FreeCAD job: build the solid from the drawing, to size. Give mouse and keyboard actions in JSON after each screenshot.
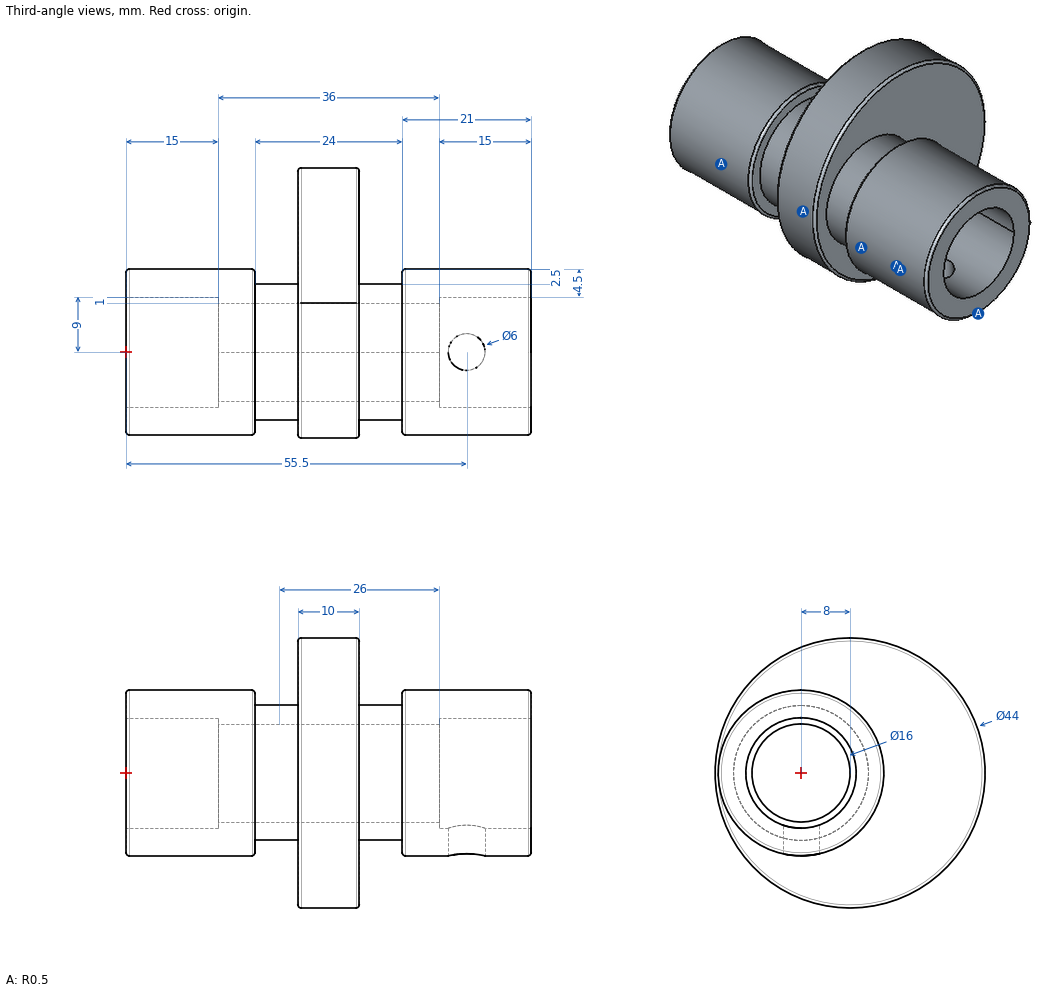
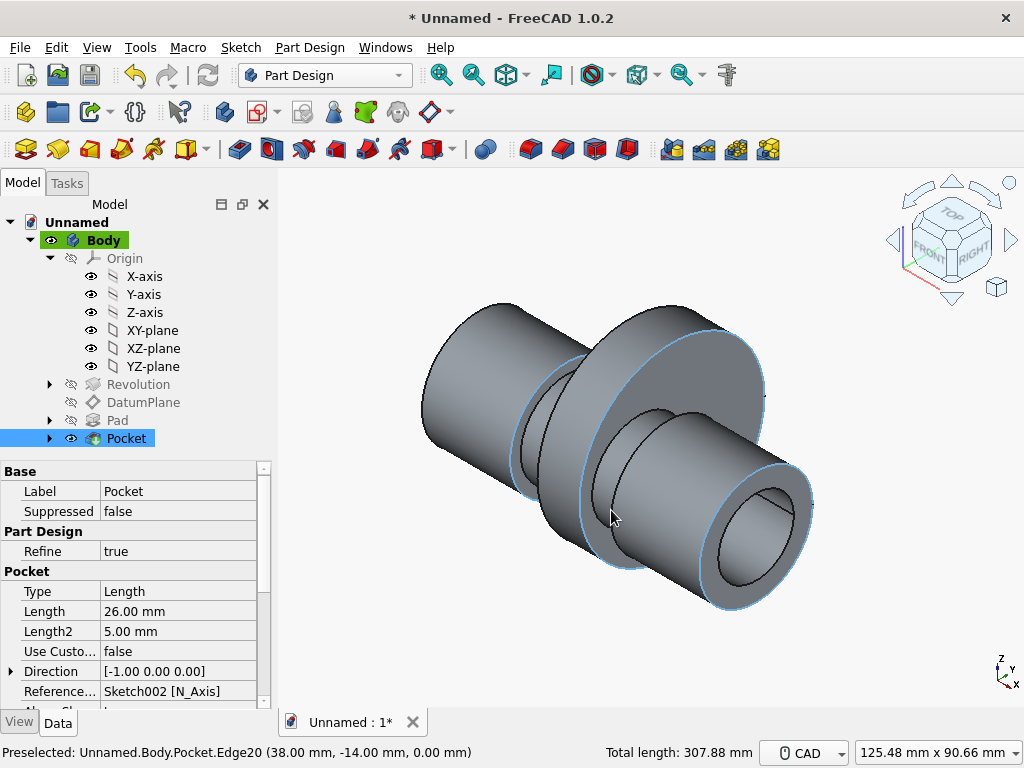
{"action": "left_click", "coordinate": [601, 339], "text": "ctrl"}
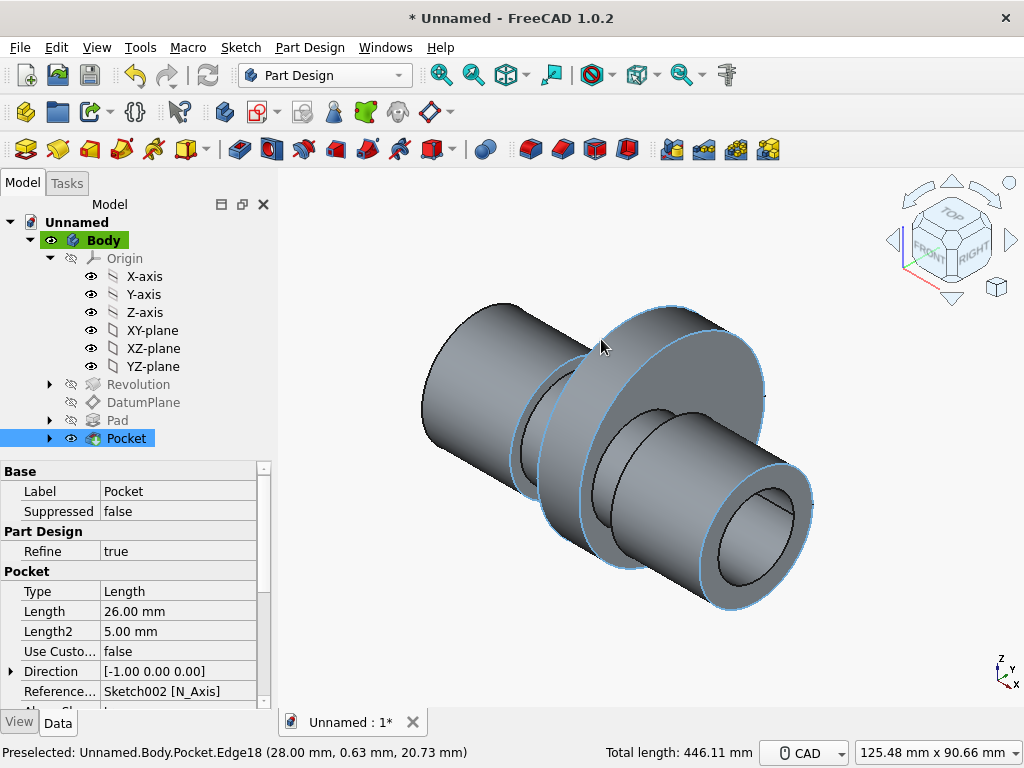
{"action": "key", "text": "2"}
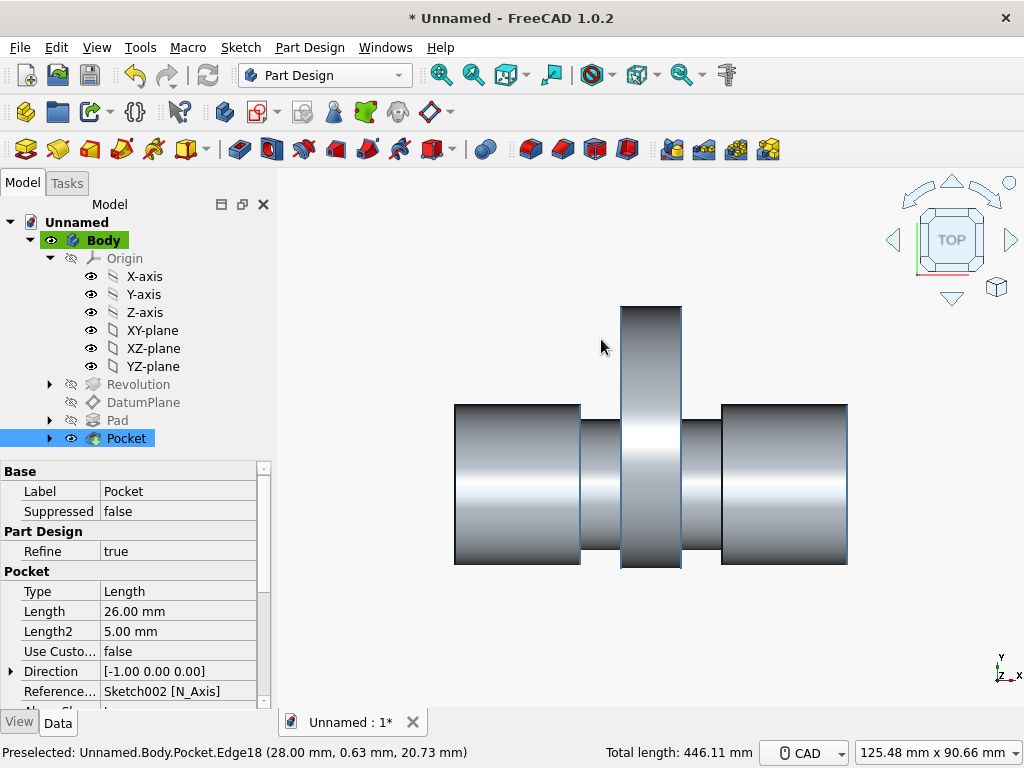
{"action": "left_click", "coordinate": [722, 549], "text": "ctrl"}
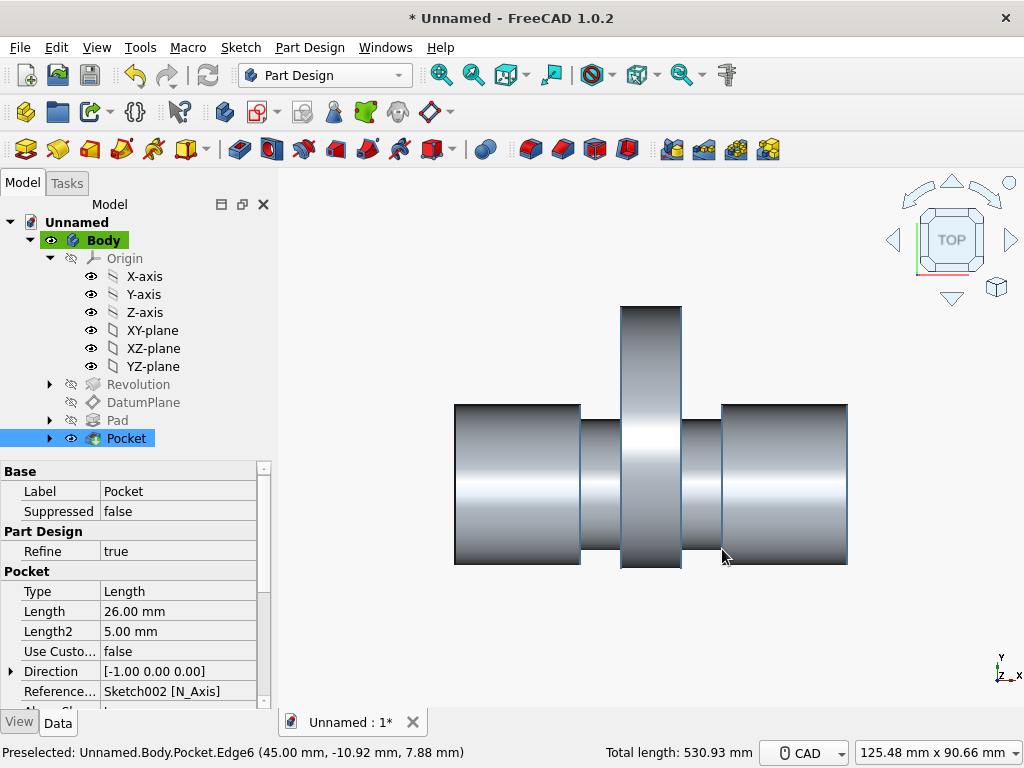
{"action": "left_click", "coordinate": [455, 549], "text": "ctrl"}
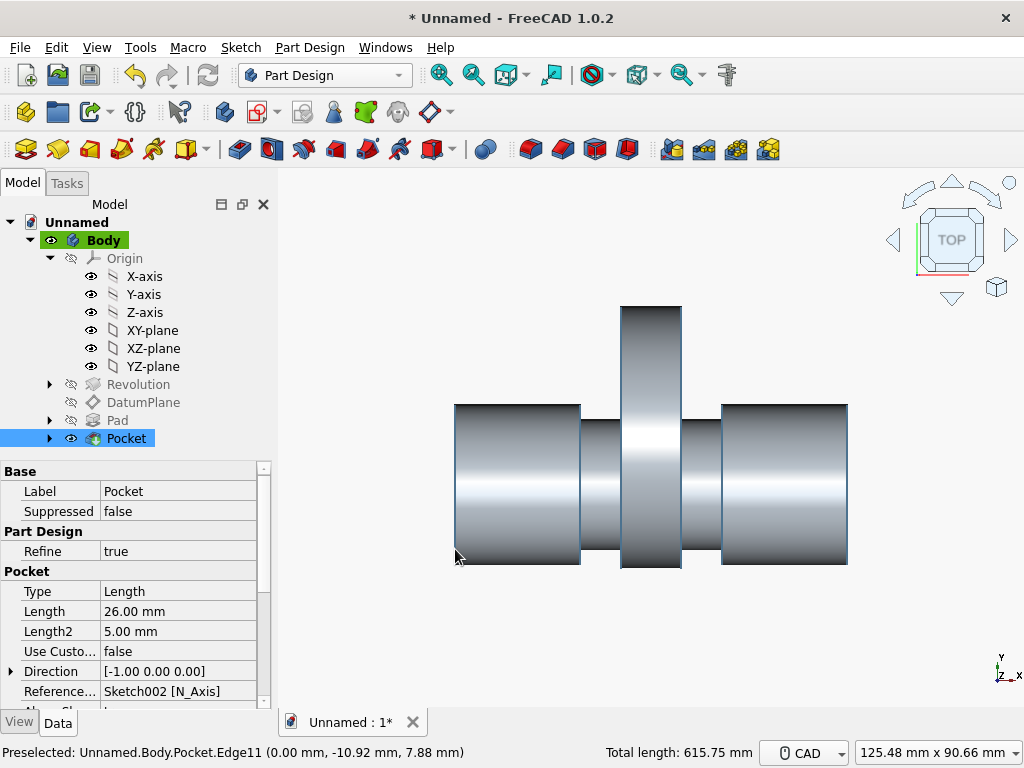
{"action": "left_click", "coordinate": [532, 150]}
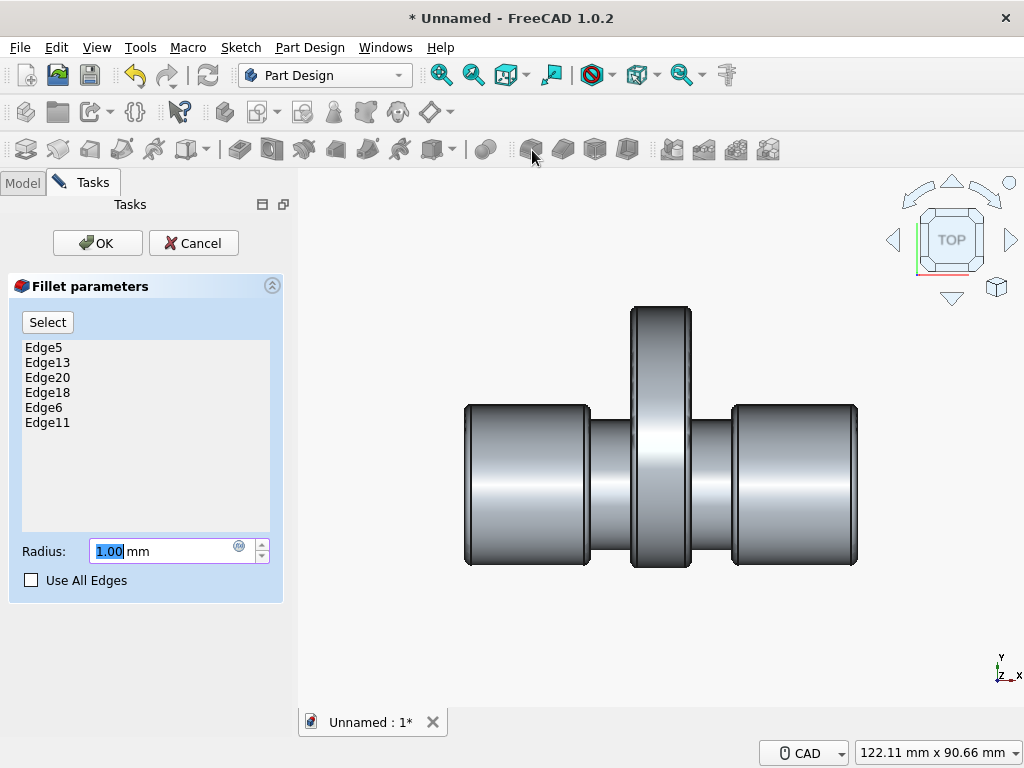
{"action": "type", "text": "0.5"}
{"action": "key", "text": "Tab"}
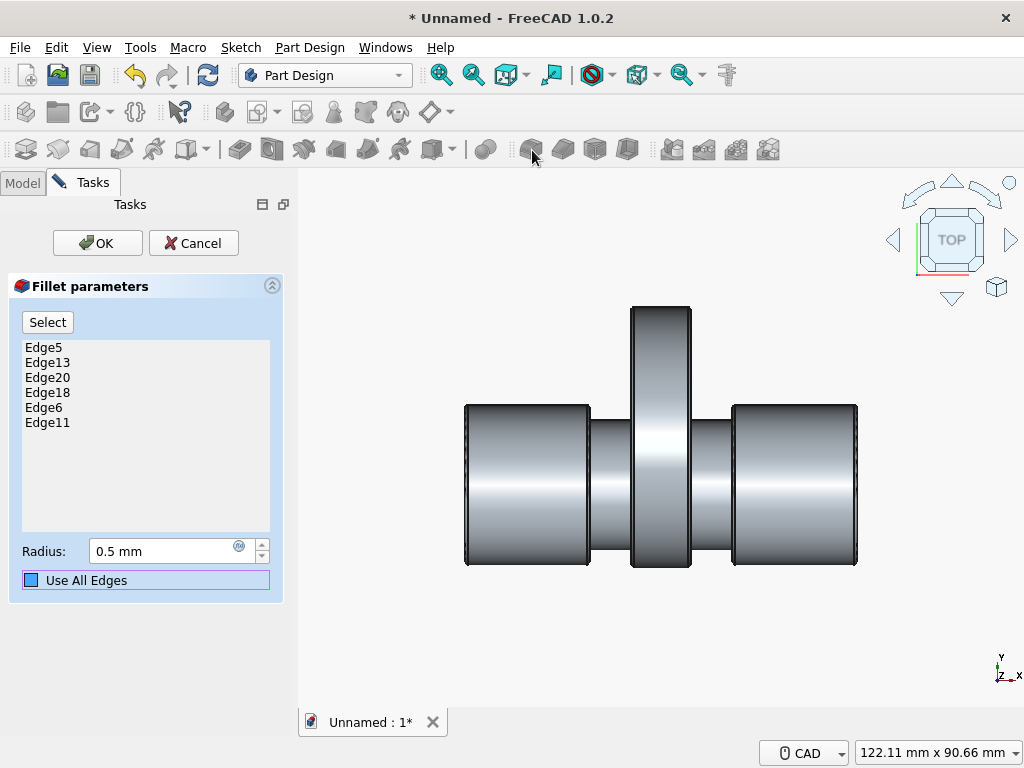
{"action": "left_click", "coordinate": [98, 243]}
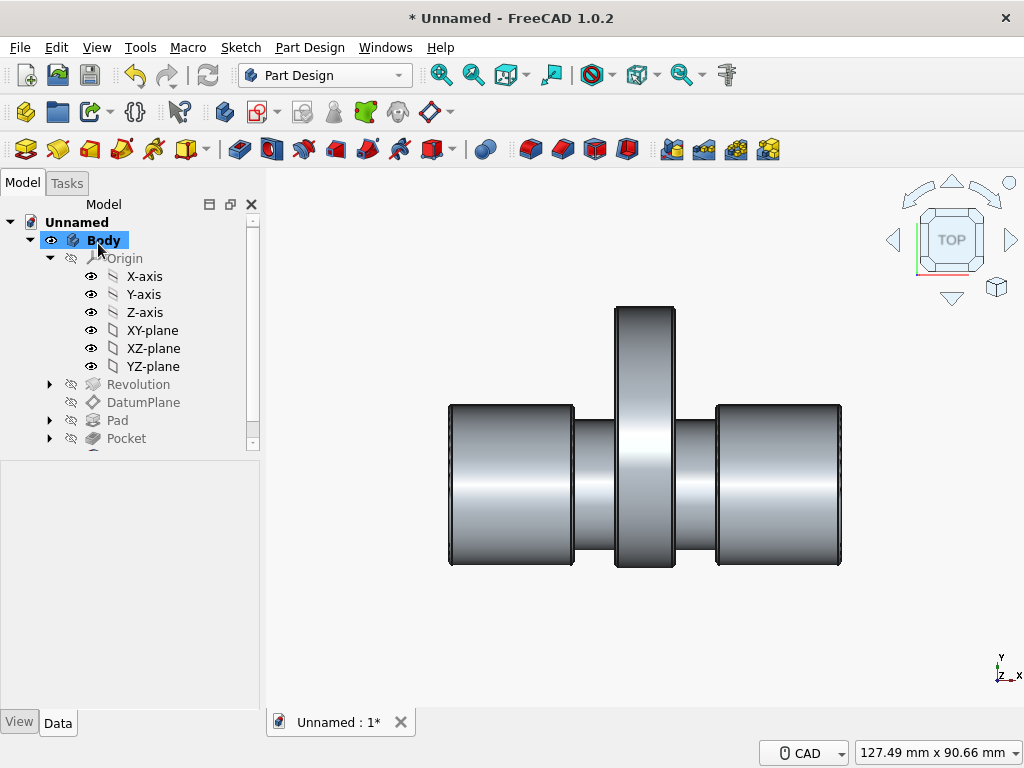
{"action": "left_click", "coordinate": [258, 112]}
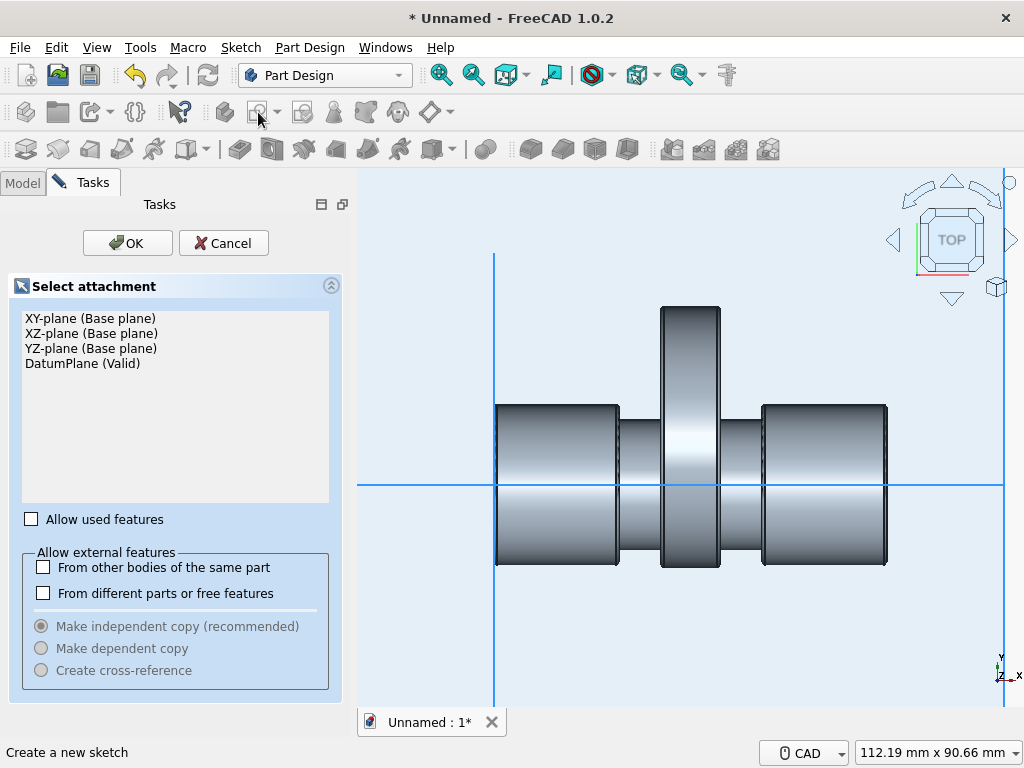
{"action": "left_click", "coordinate": [82, 318]}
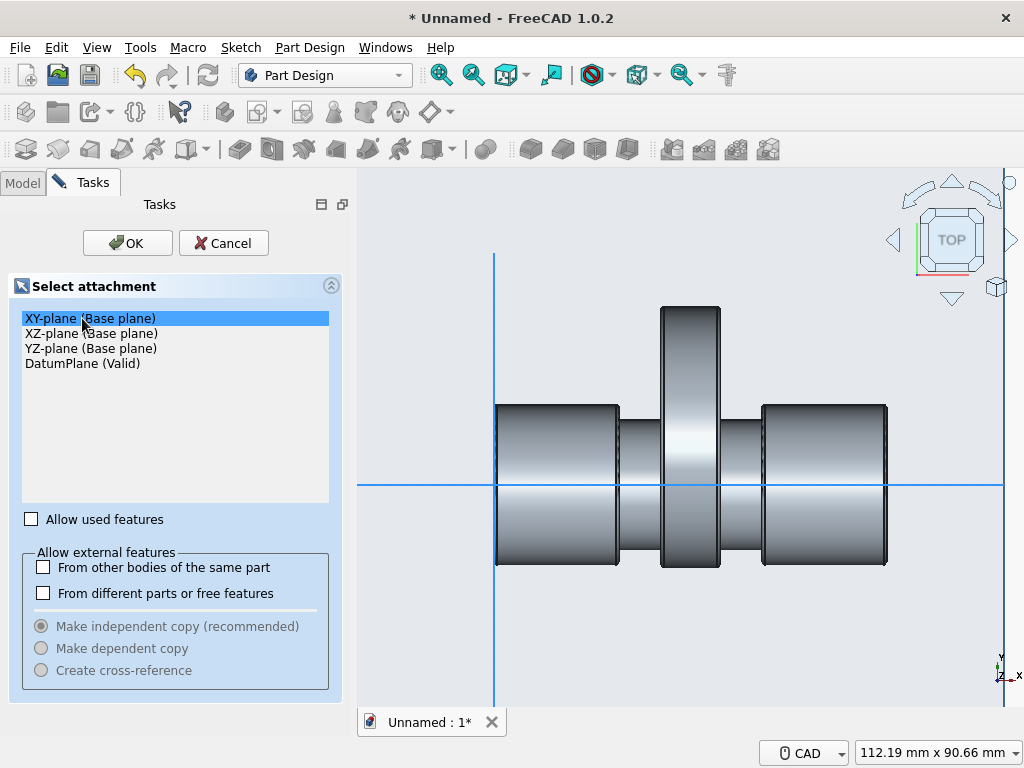
{"action": "left_click", "coordinate": [128, 243]}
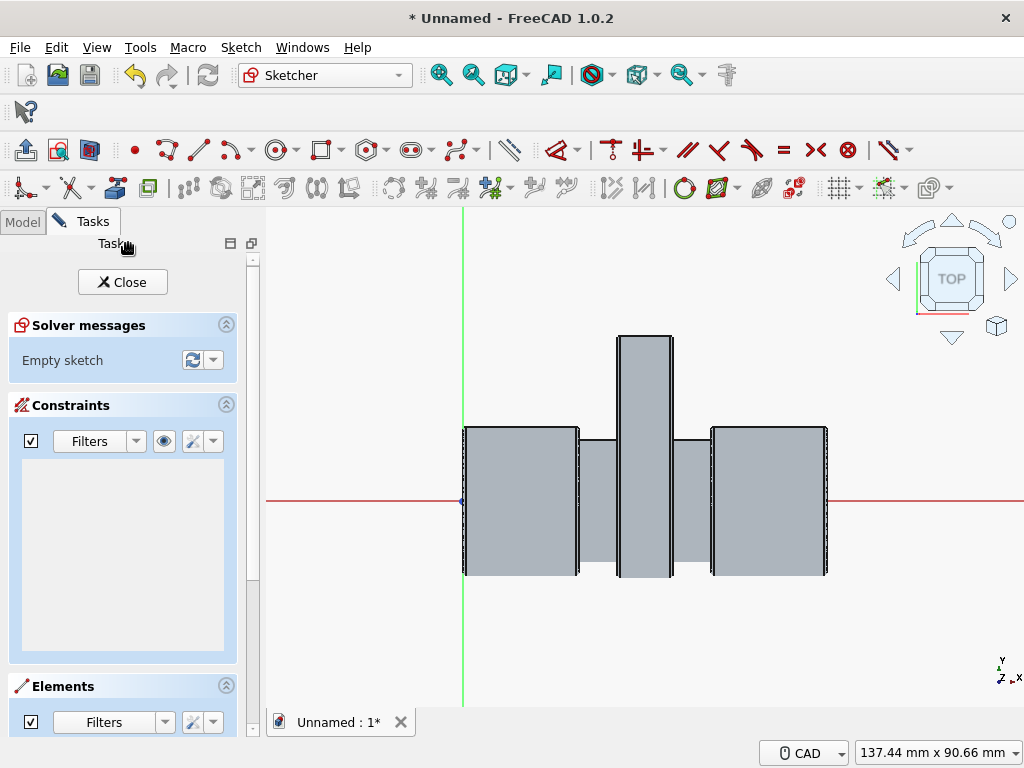
{"action": "left_click", "coordinate": [90, 150]}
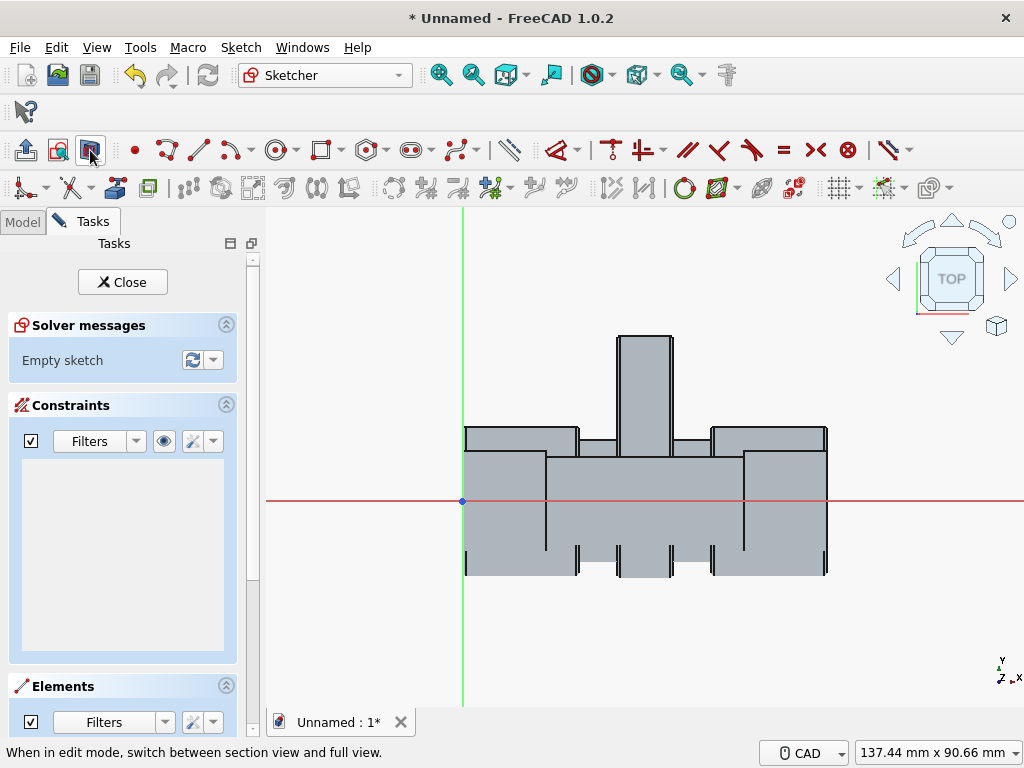
{"action": "scroll", "coordinate": [793, 507], "scroll_direction": "up", "scroll_amount": 11}